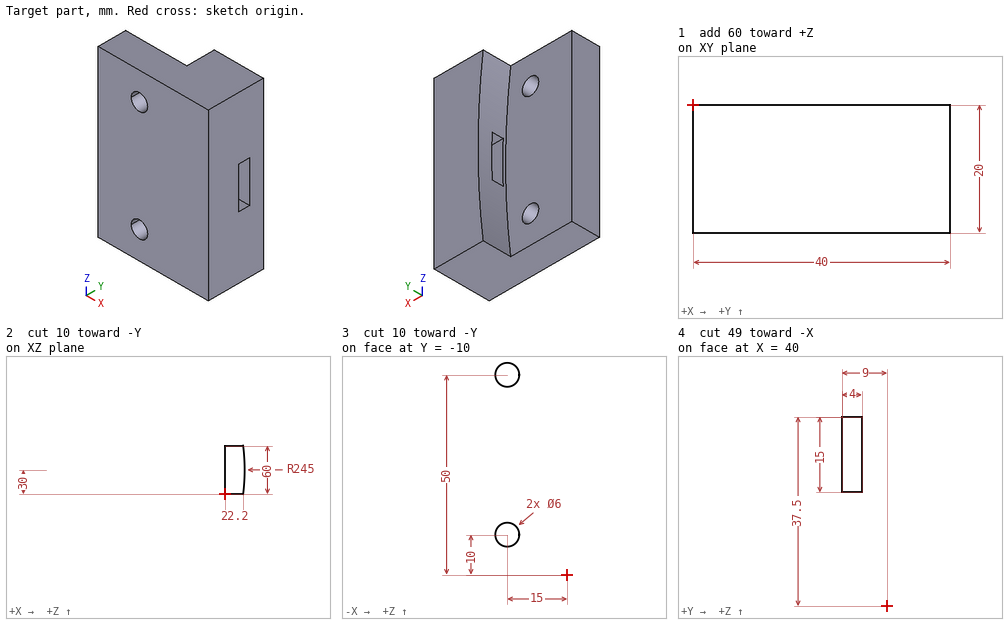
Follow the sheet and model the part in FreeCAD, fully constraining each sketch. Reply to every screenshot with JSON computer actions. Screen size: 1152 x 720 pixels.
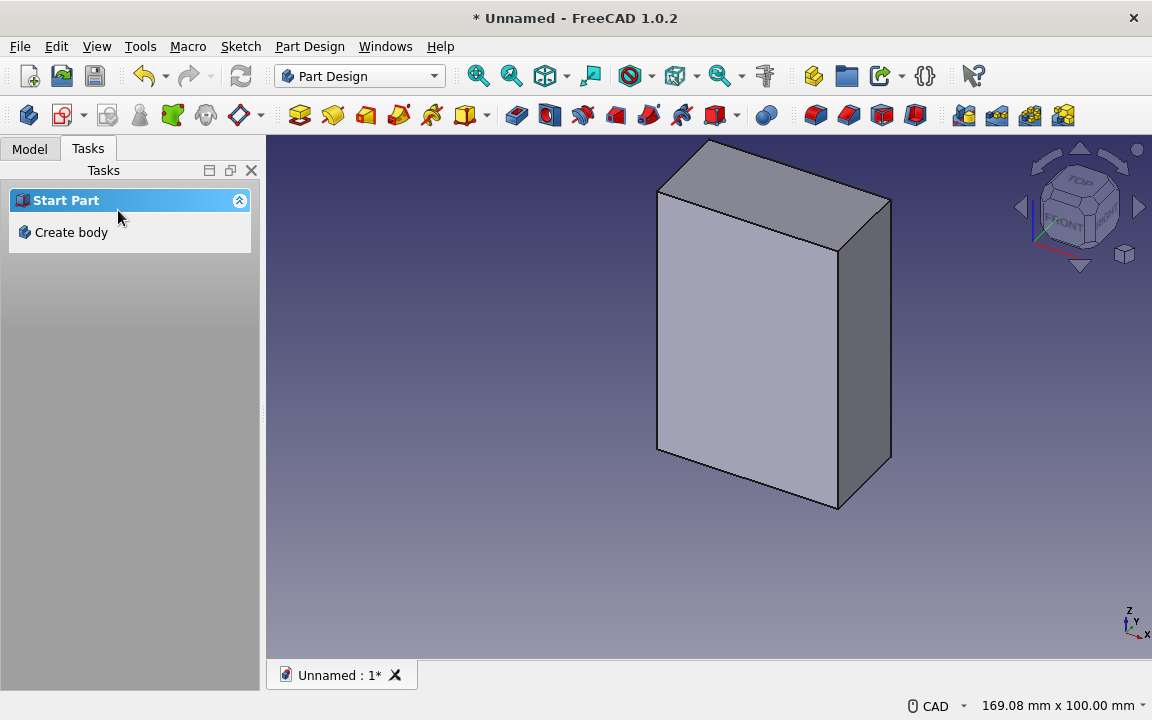
{"action": "left_click", "coordinate": [62, 116]}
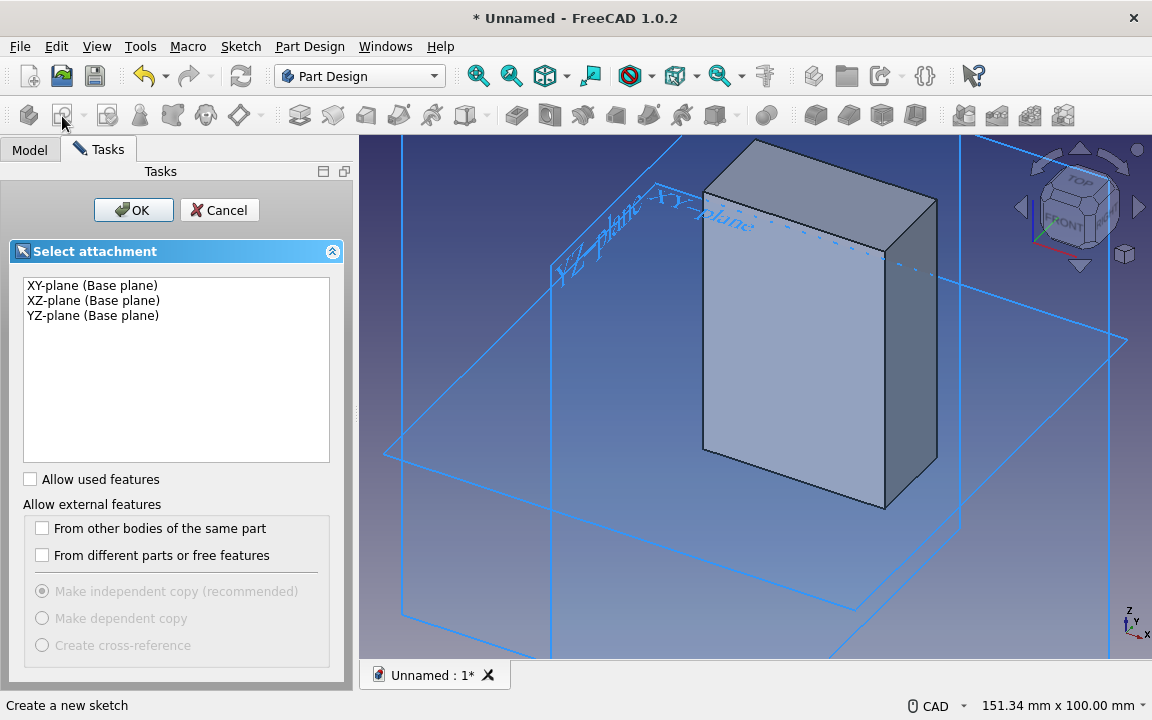
{"action": "left_click", "coordinate": [84, 300]}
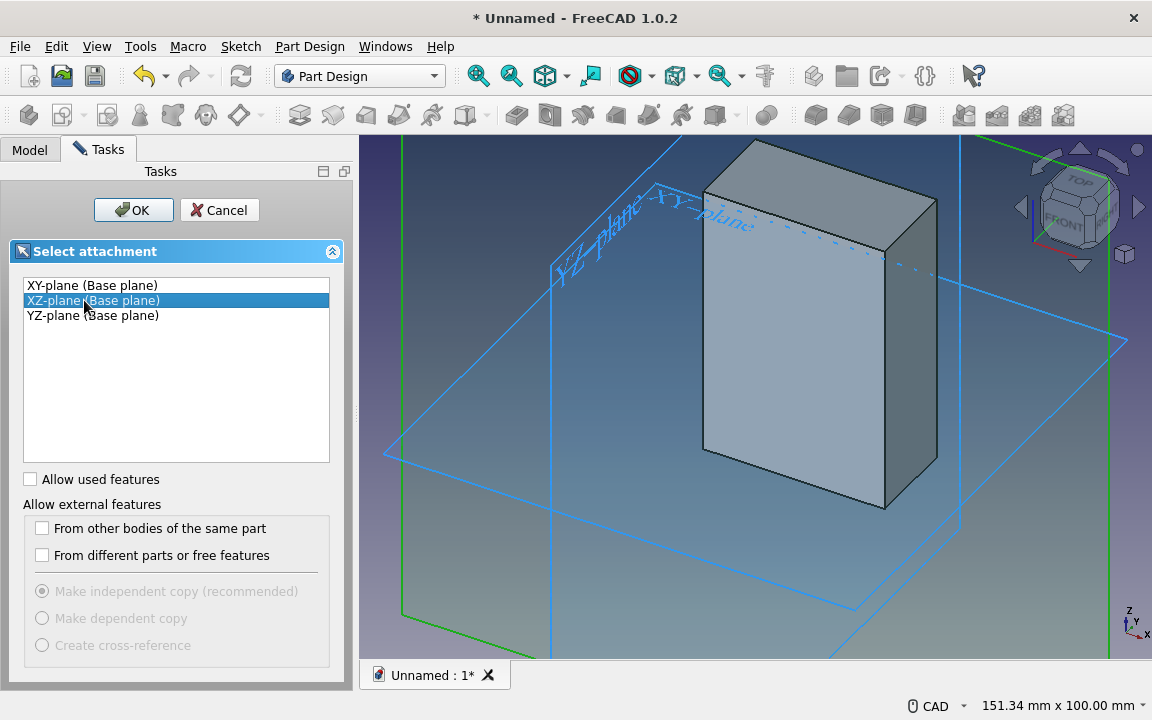
{"action": "left_click", "coordinate": [134, 210]}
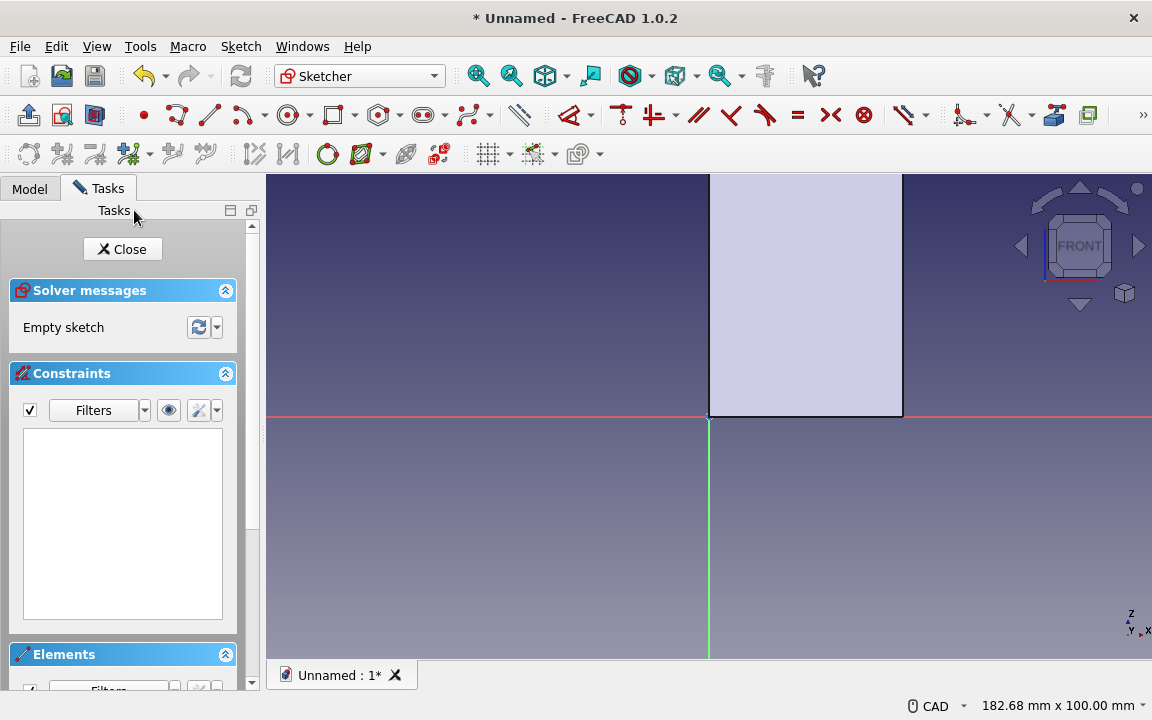
{"action": "left_click", "coordinate": [95, 116]}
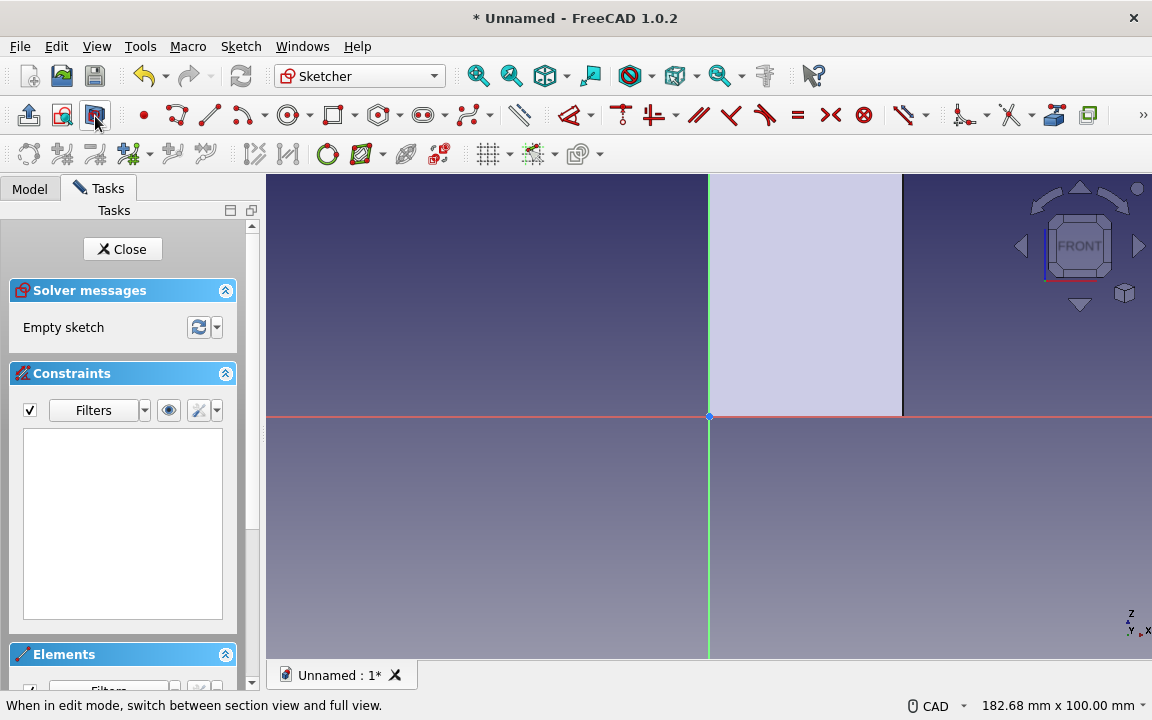
{"action": "scroll", "coordinate": [383, 631], "scroll_direction": "down", "scroll_amount": 2}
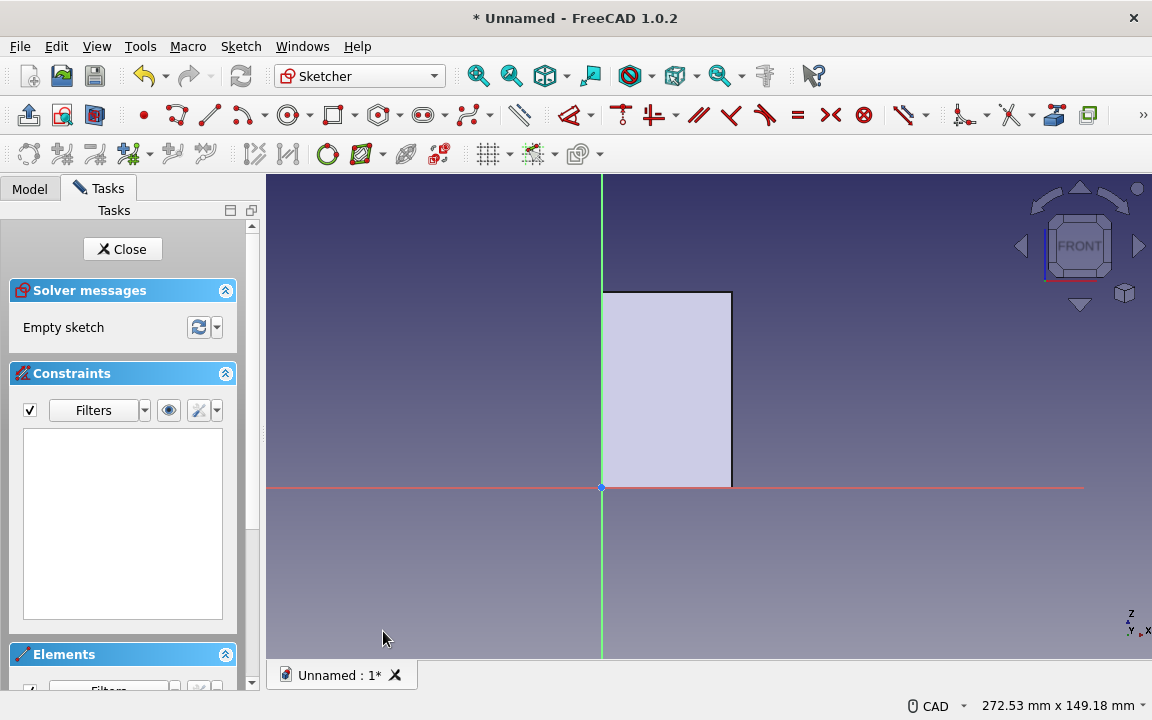
{"action": "scroll", "coordinate": [641, 336], "scroll_direction": "up", "scroll_amount": 2}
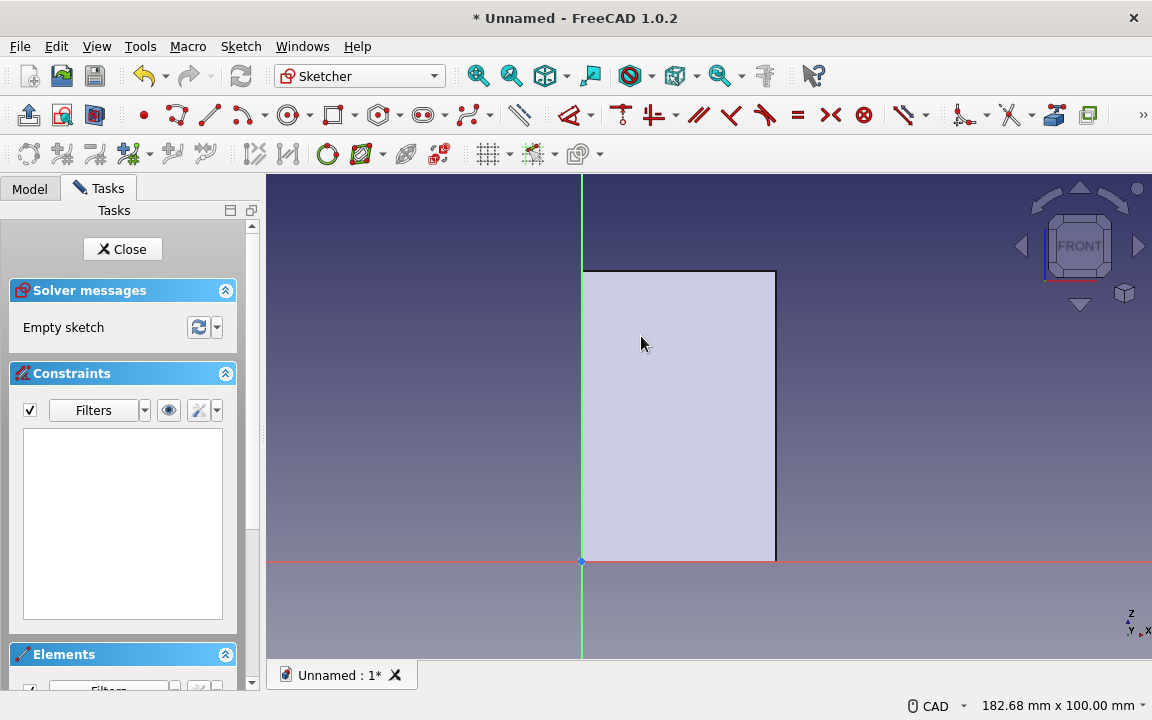
{"action": "key", "text": "g m"}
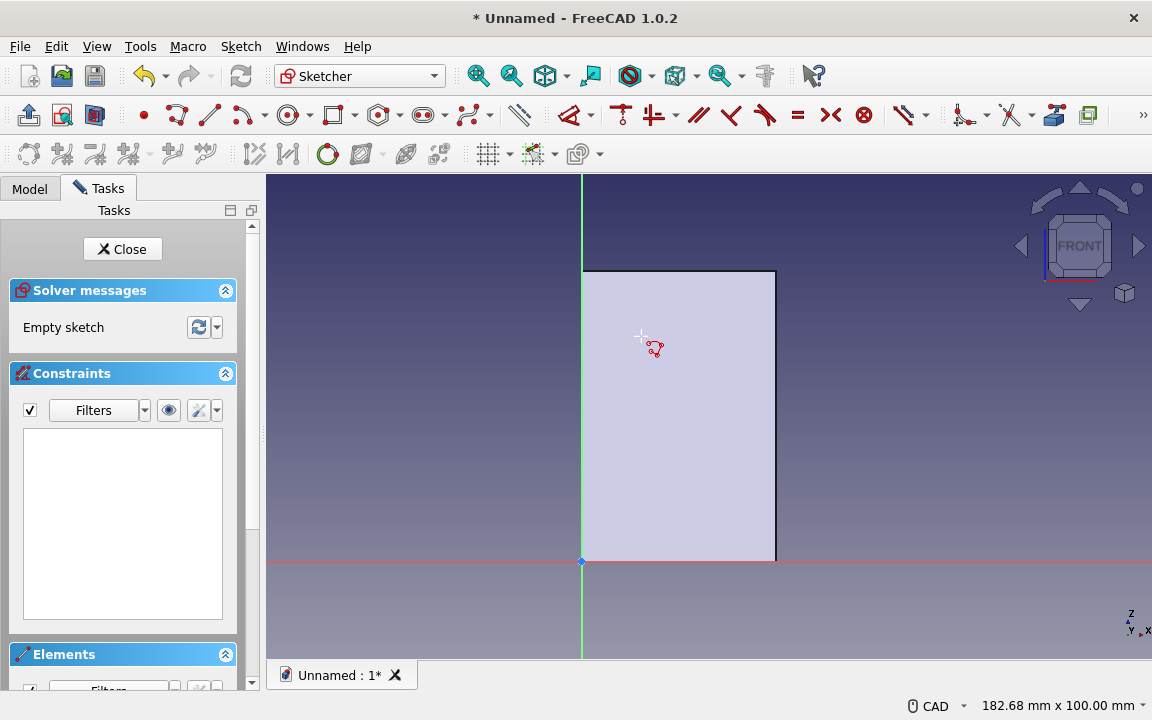
{"action": "left_click", "coordinate": [690, 562]}
{"action": "left_click", "coordinate": [582, 562]}
{"action": "left_click", "coordinate": [591, 271]}
{"action": "left_click", "coordinate": [690, 271]}
{"action": "right_click", "coordinate": [690, 271]}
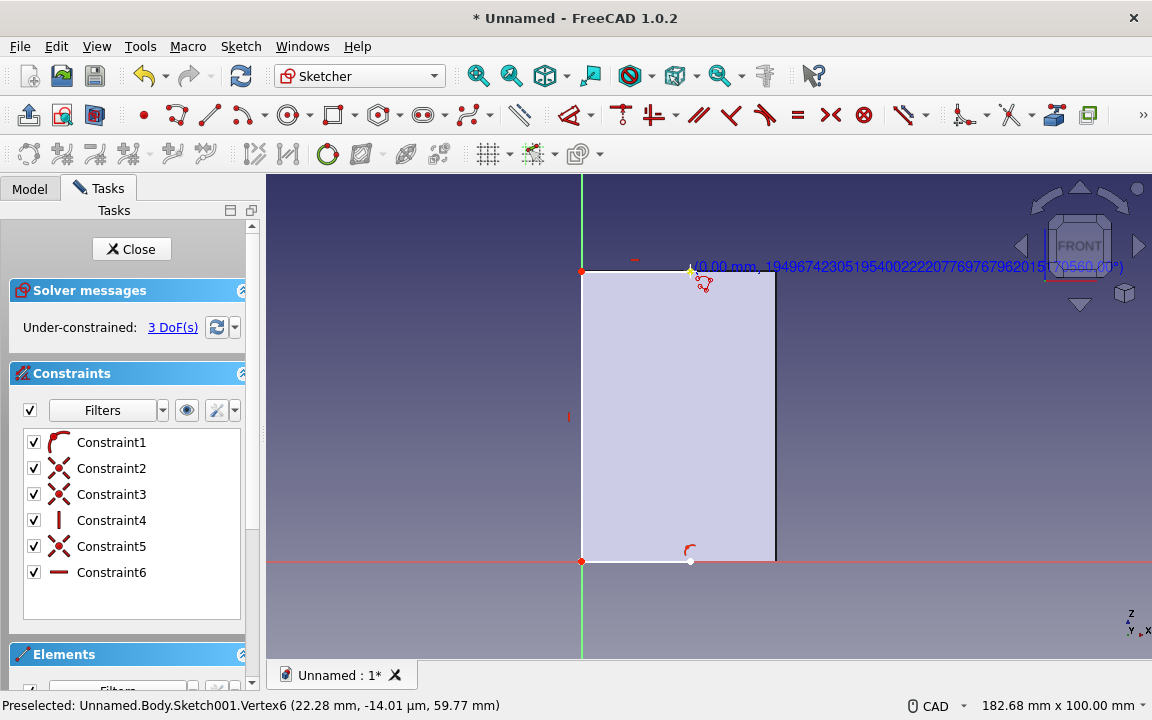
{"action": "left_click", "coordinate": [264, 116]}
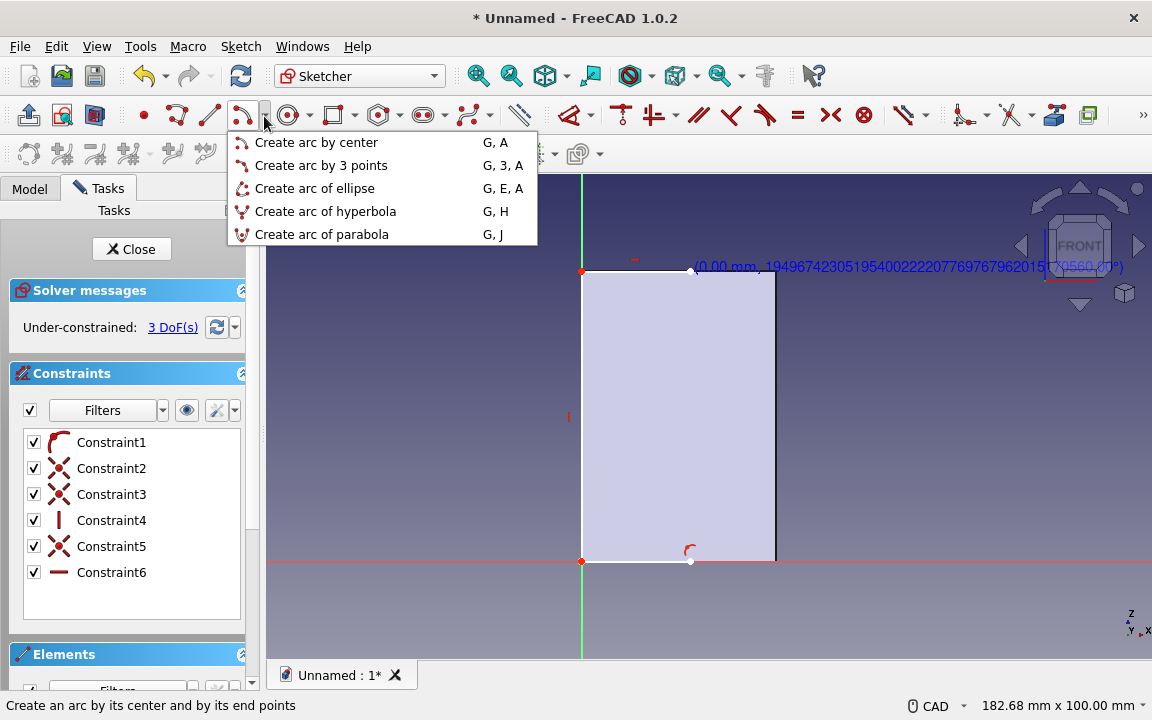
{"action": "left_click", "coordinate": [382, 166]}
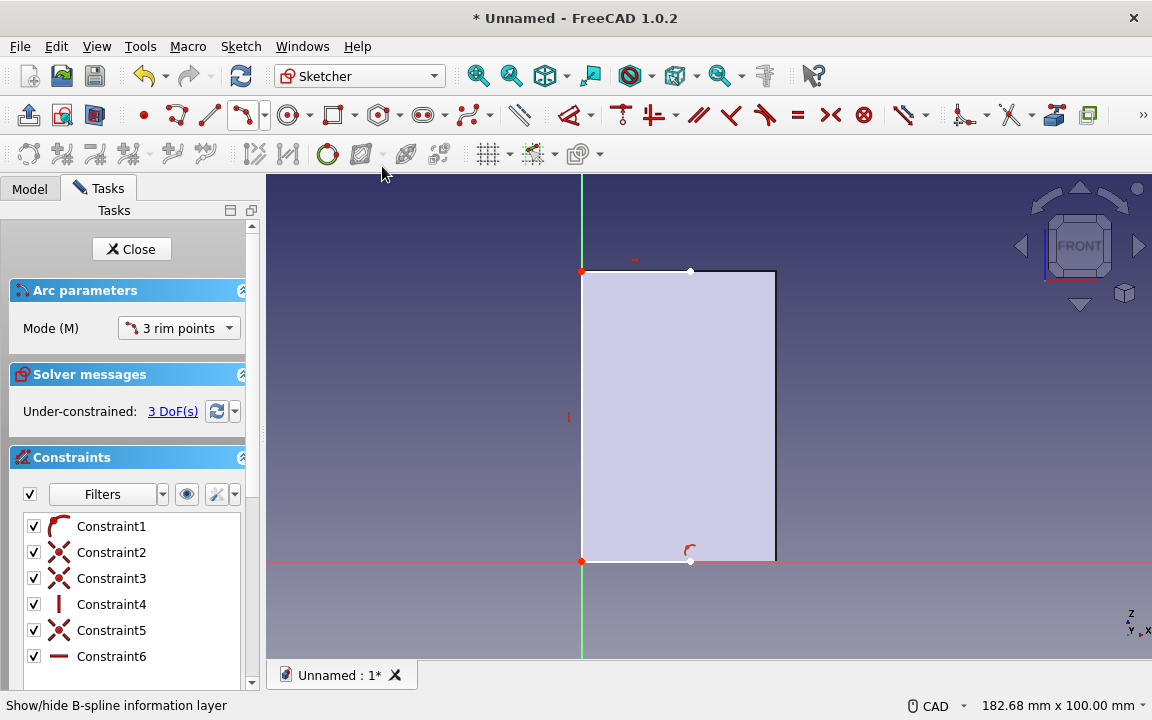
{"action": "left_click", "coordinate": [690, 272]}
{"action": "left_click", "coordinate": [690, 562]}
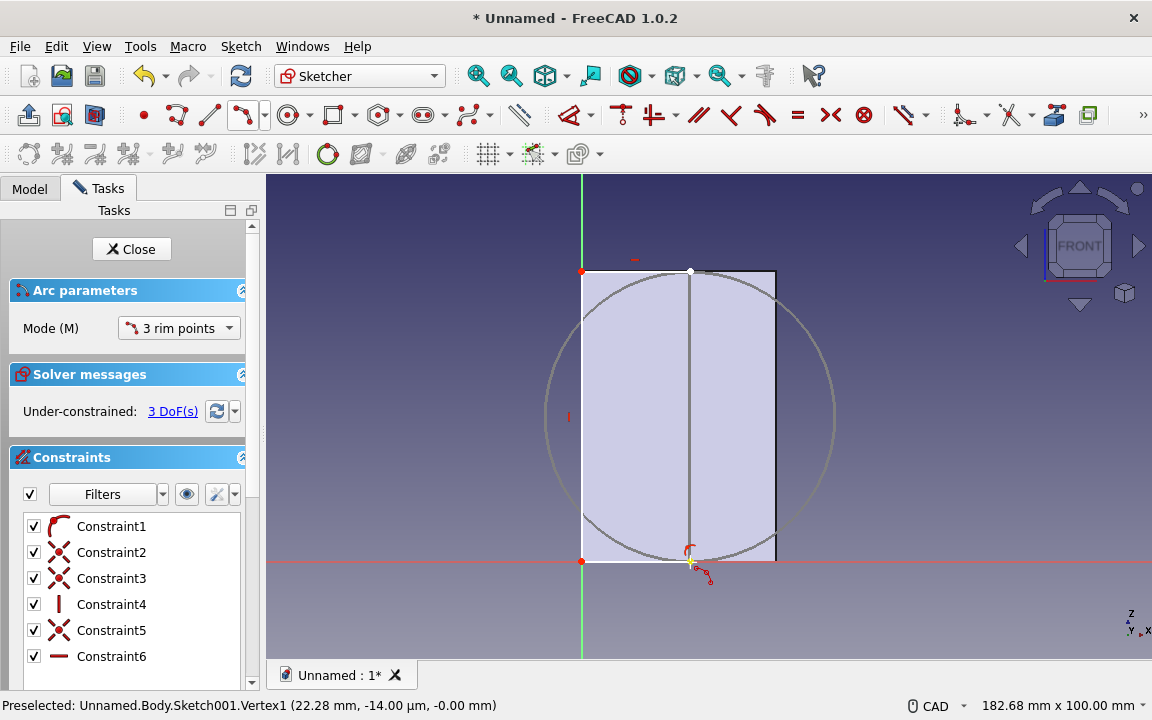
{"action": "scroll", "coordinate": [699, 416], "scroll_direction": "up", "scroll_amount": 3}